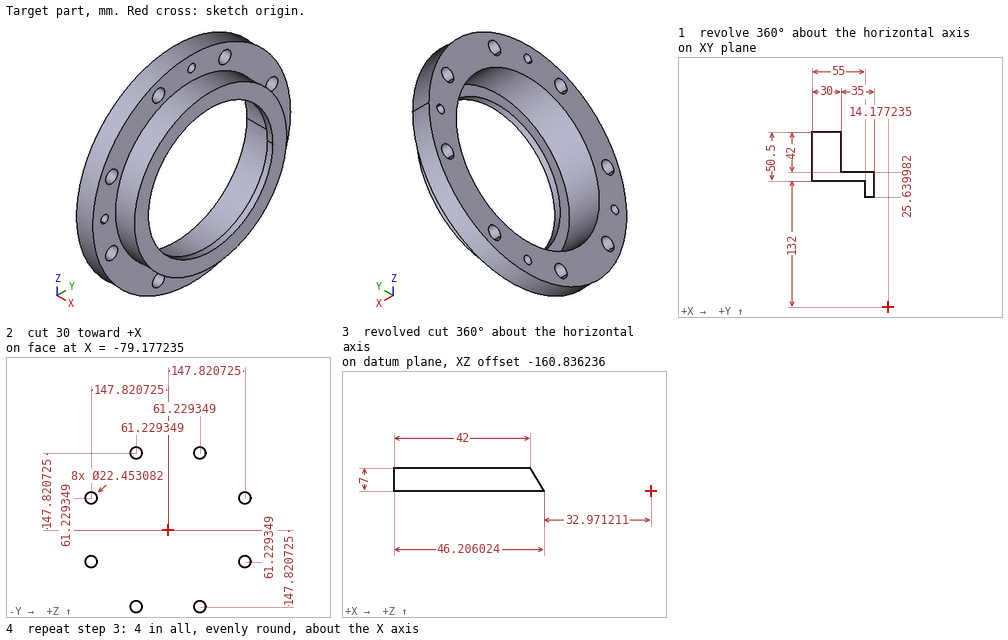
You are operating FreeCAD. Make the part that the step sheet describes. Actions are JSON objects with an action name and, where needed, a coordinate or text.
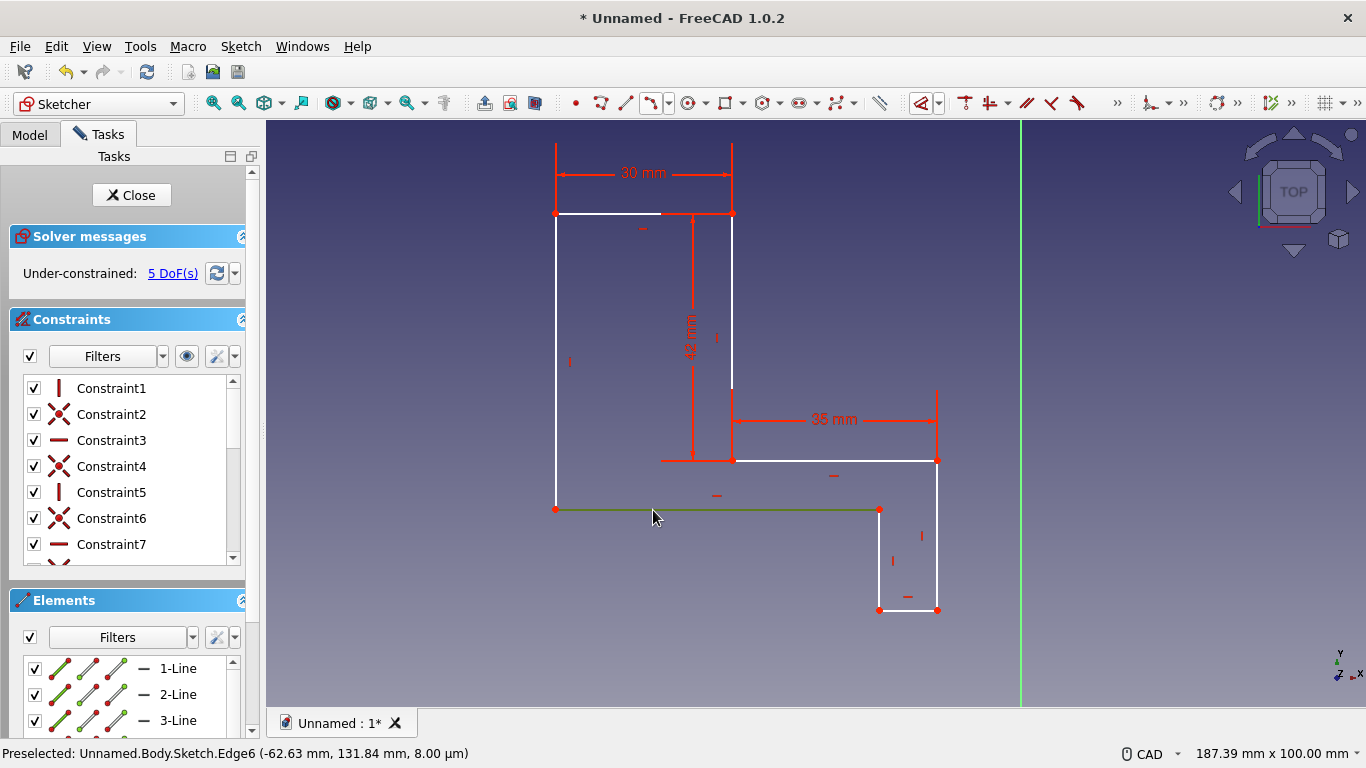
{"action": "key", "text": "l"}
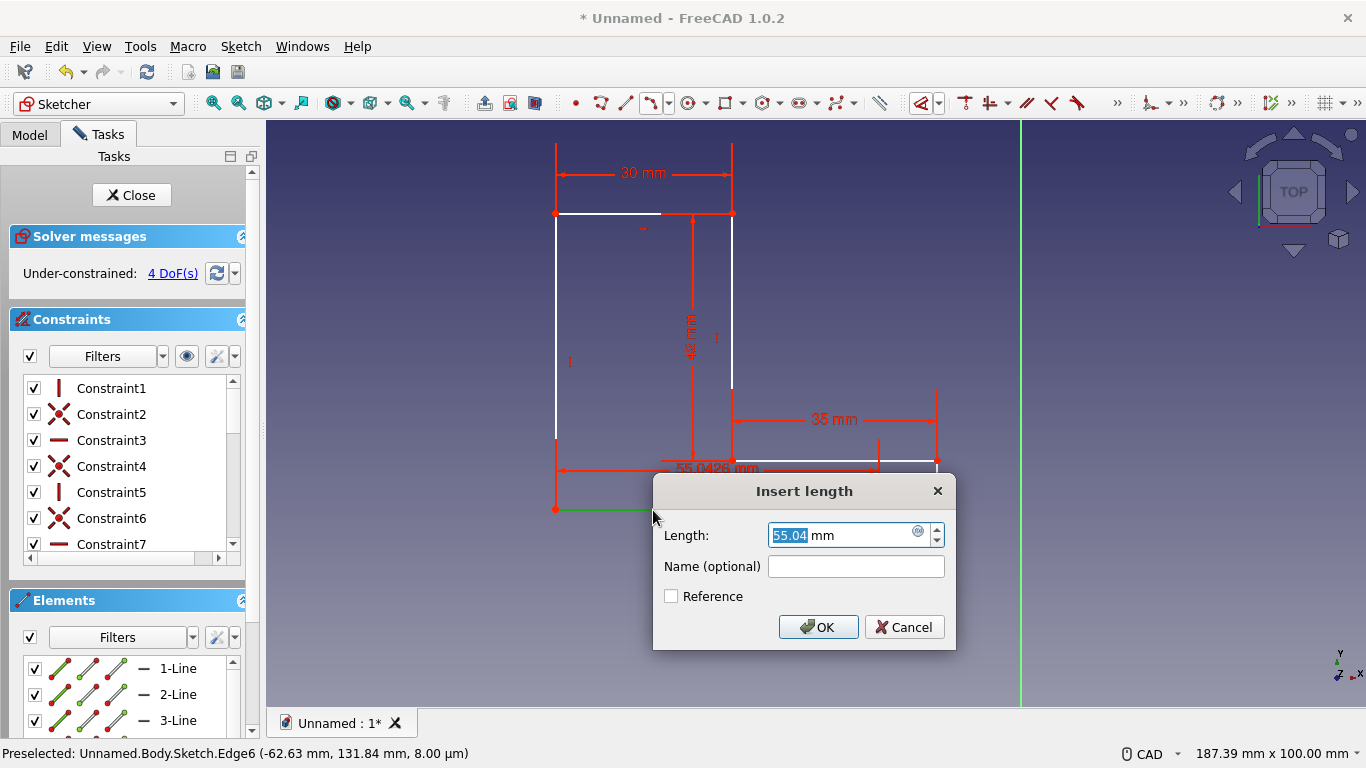
{"action": "type", "text": "55"}
{"action": "key", "text": "Return"}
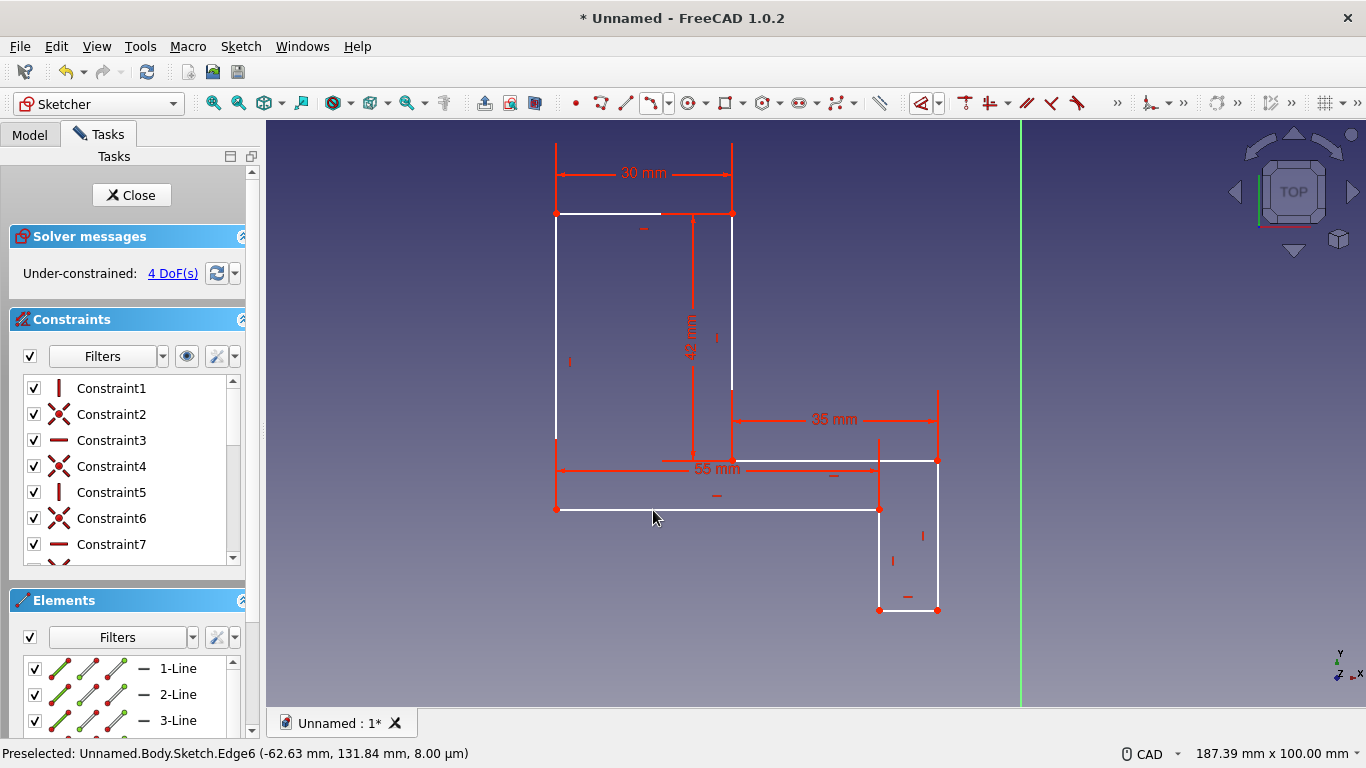
{"action": "left_click", "coordinate": [556, 303]}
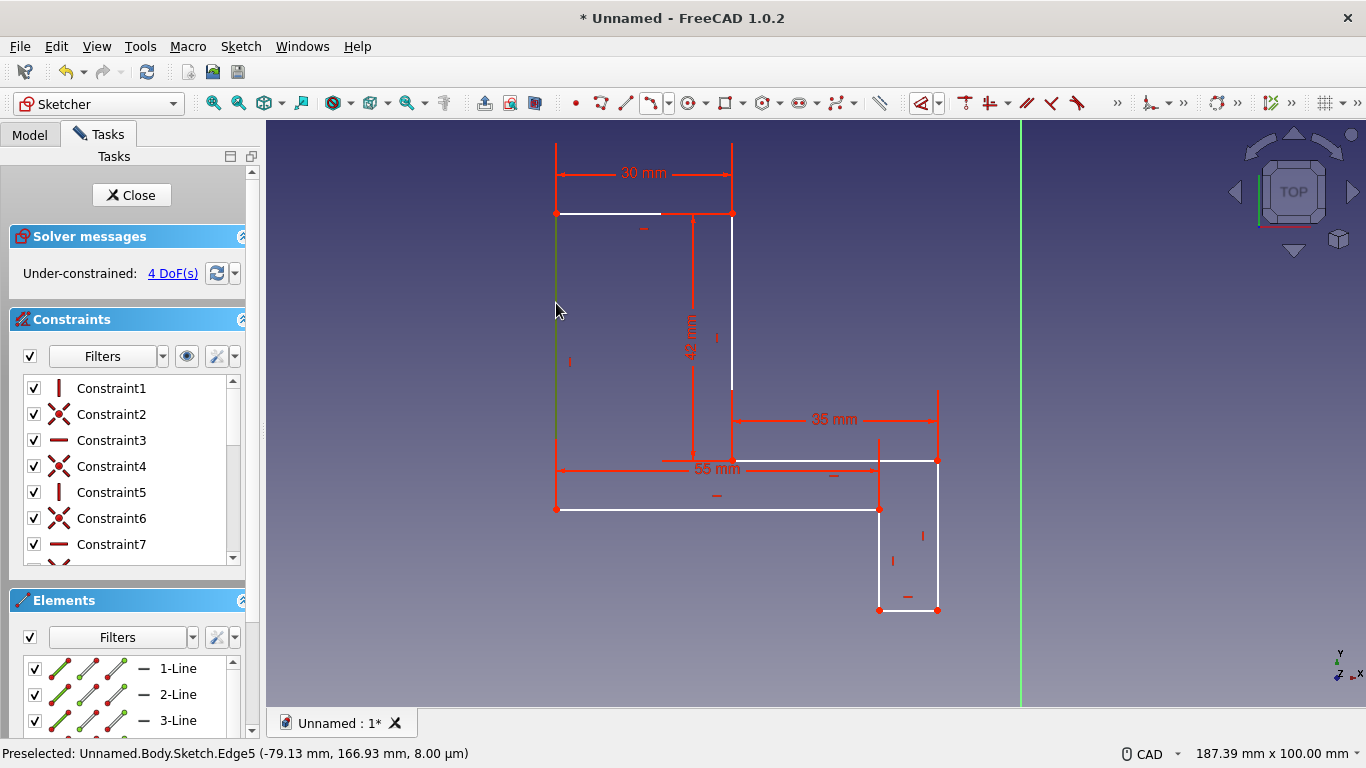
{"action": "key", "text": "i"}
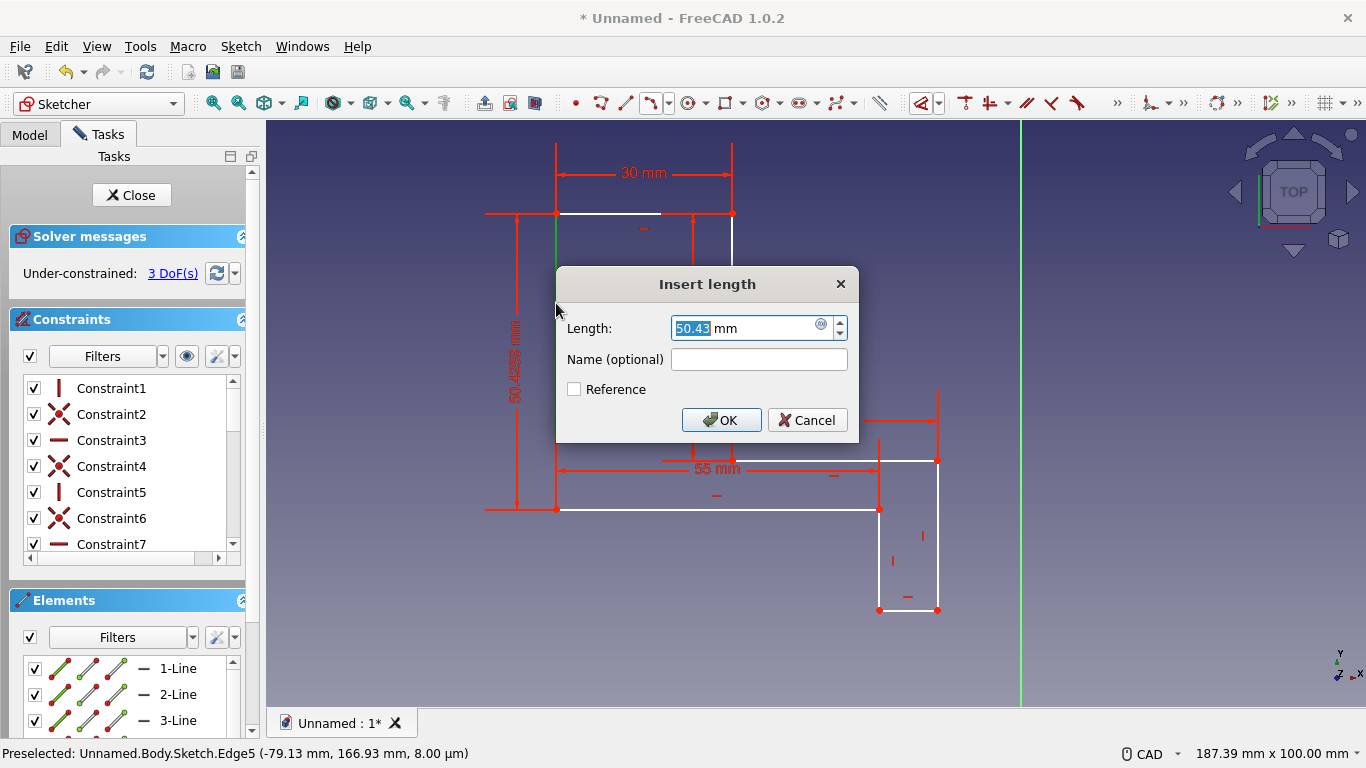
{"action": "type", "text": "50.5"}
{"action": "key", "text": "Return"}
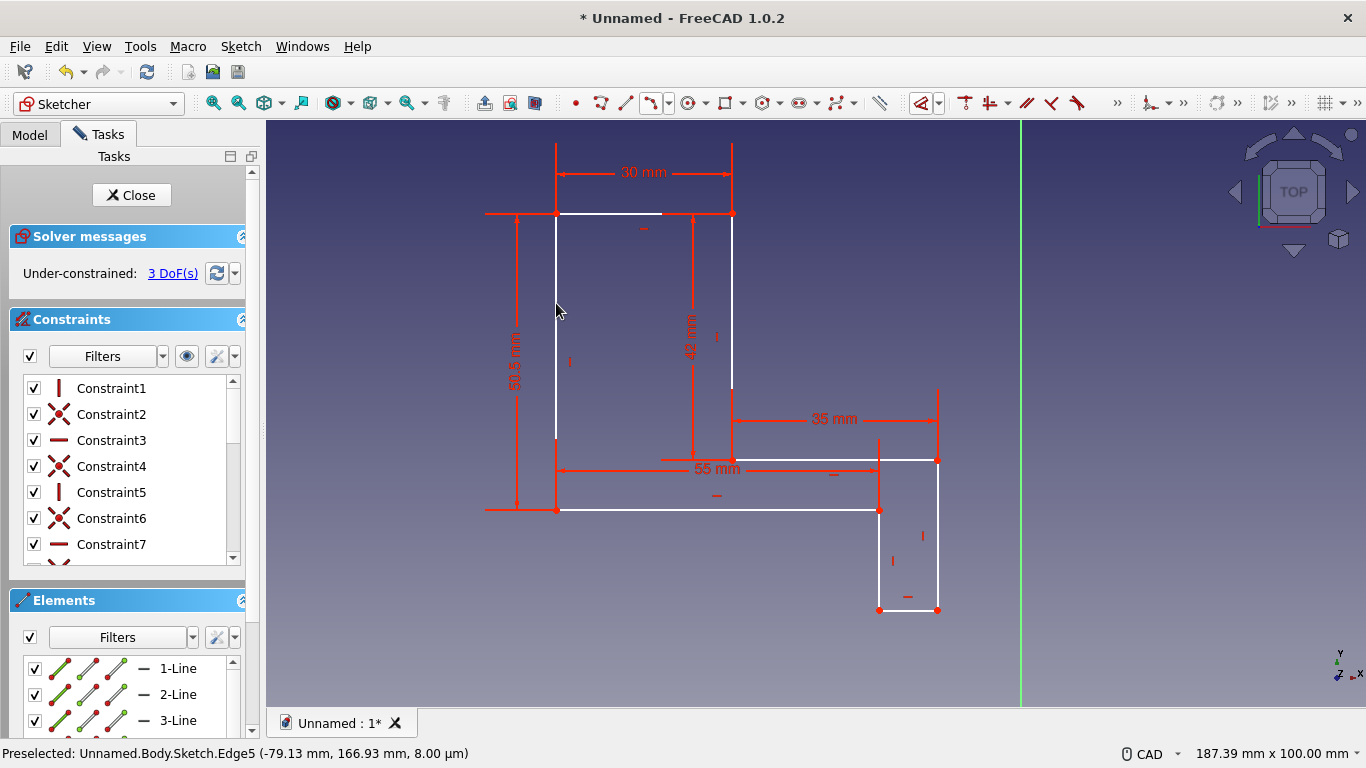
{"action": "left_click", "coordinate": [556, 510]}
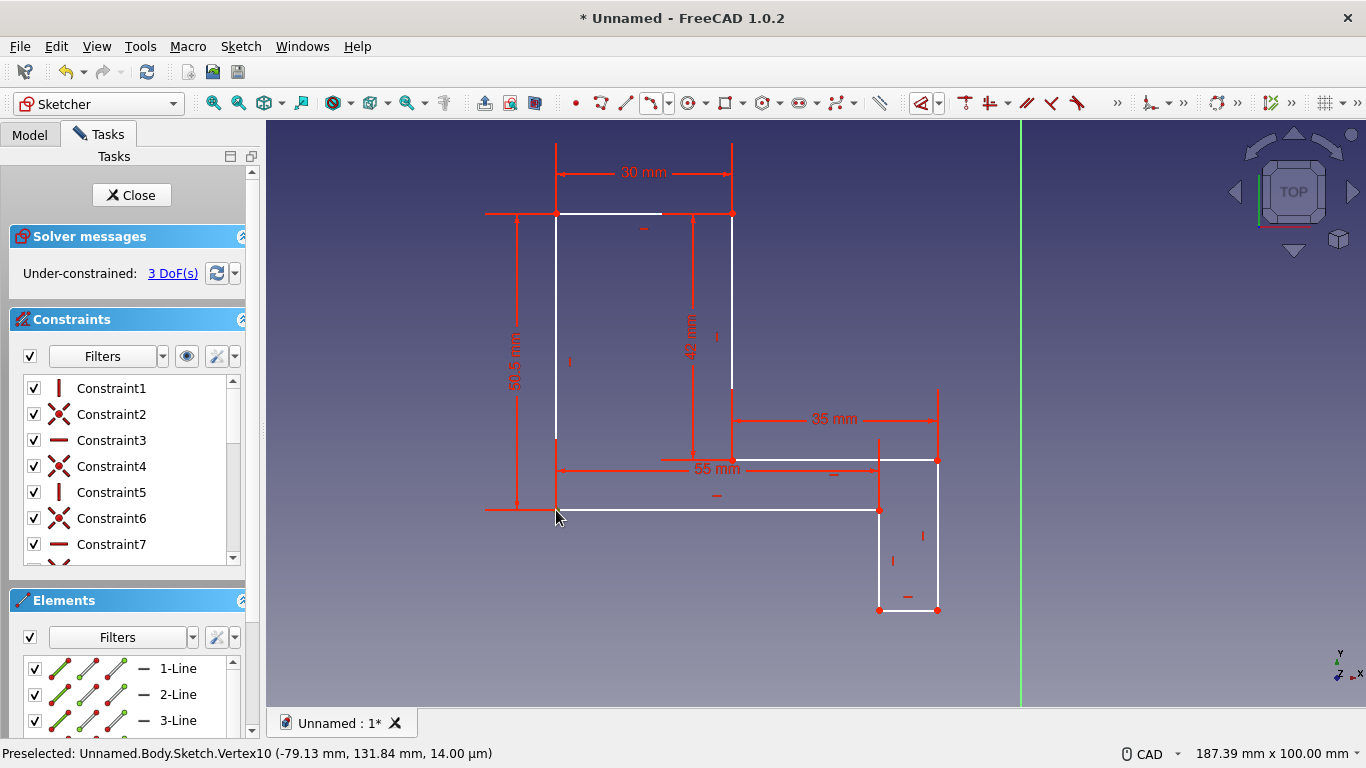
{"action": "key", "text": "i"}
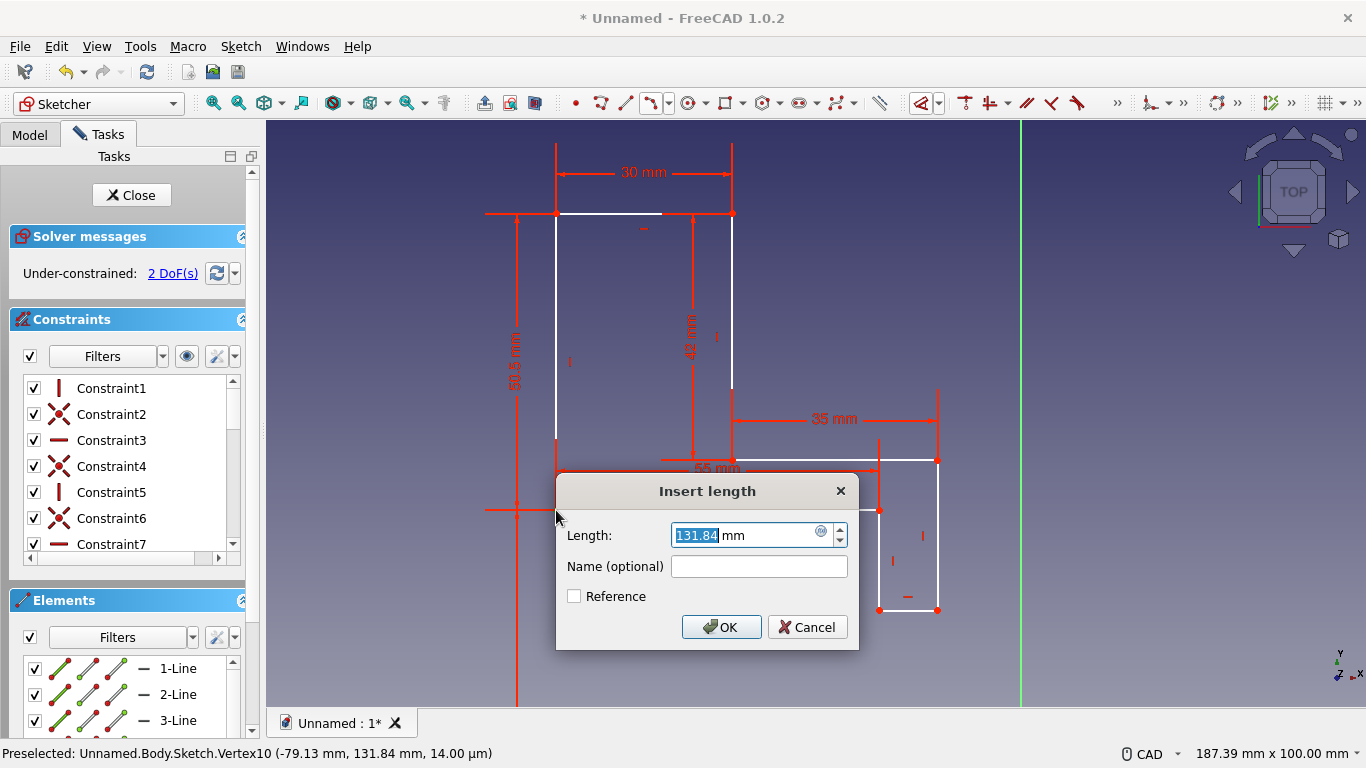
{"action": "type", "text": "132"}
{"action": "key", "text": "Return"}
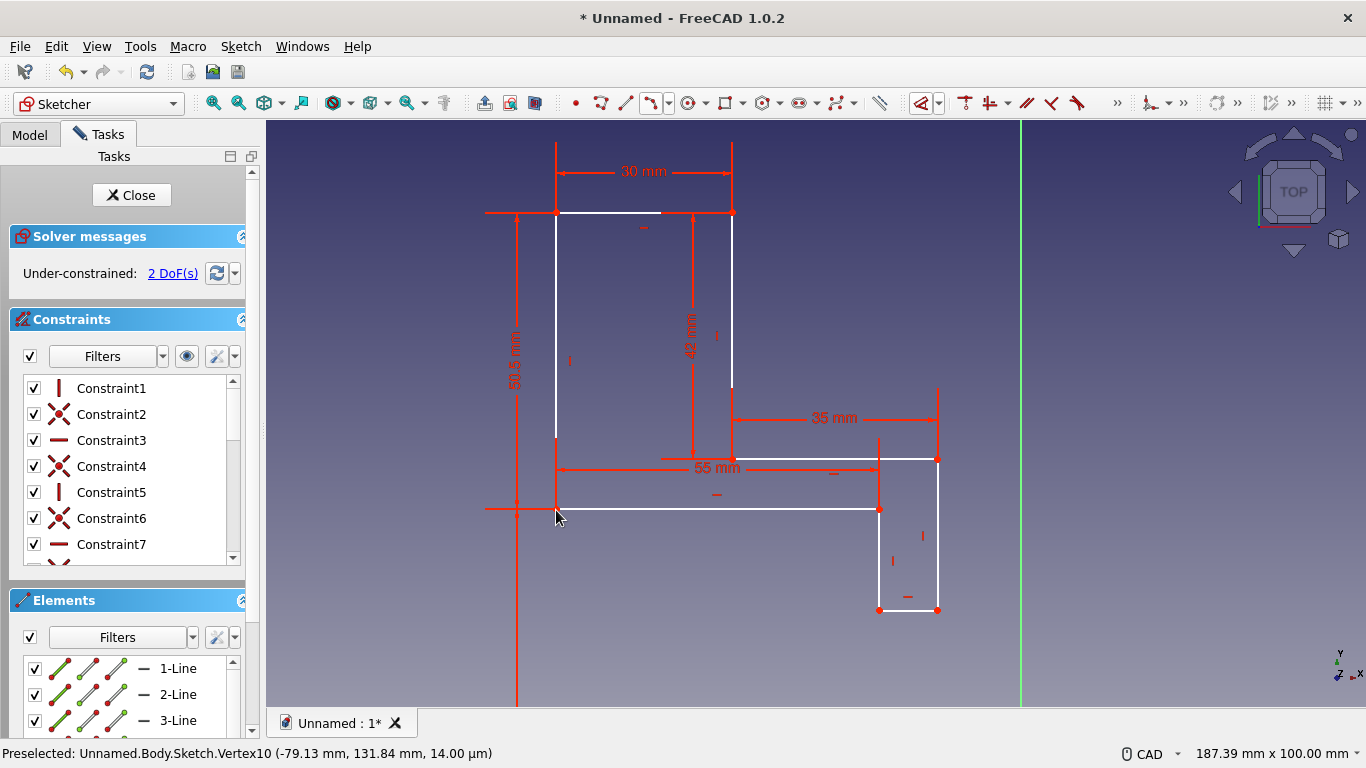
{"action": "left_click", "coordinate": [938, 565]}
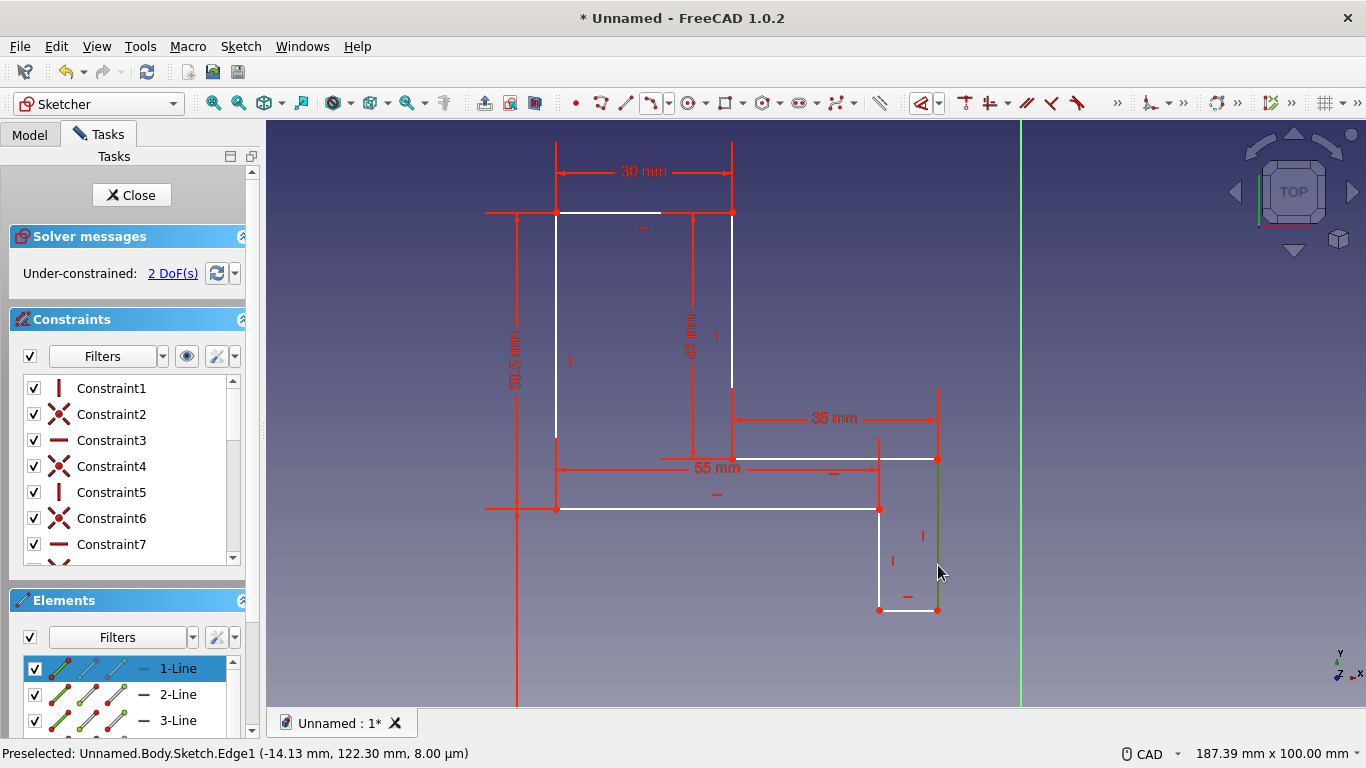
{"action": "left_click", "coordinate": [938, 104]}